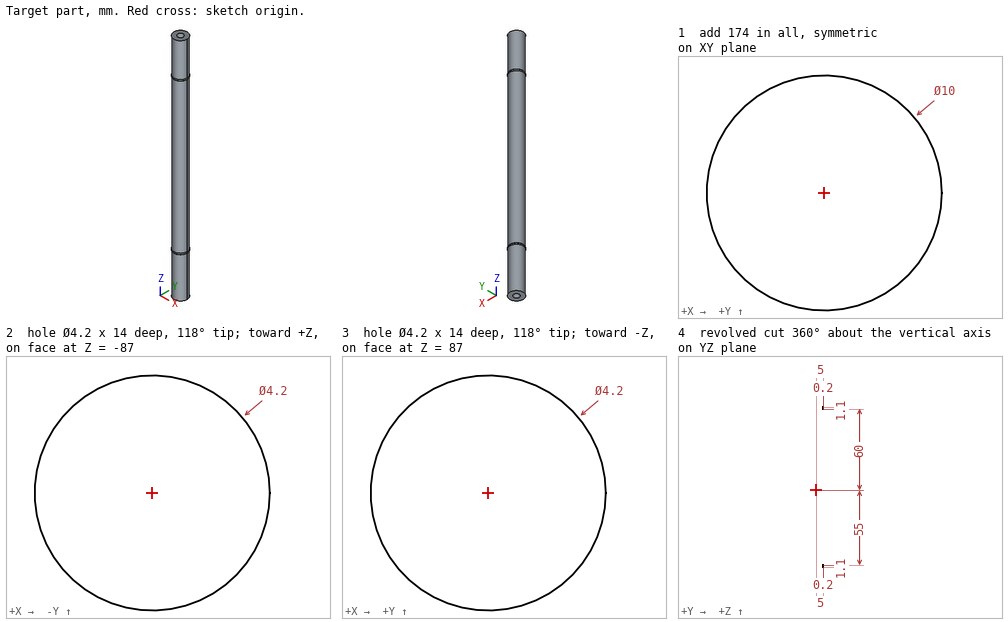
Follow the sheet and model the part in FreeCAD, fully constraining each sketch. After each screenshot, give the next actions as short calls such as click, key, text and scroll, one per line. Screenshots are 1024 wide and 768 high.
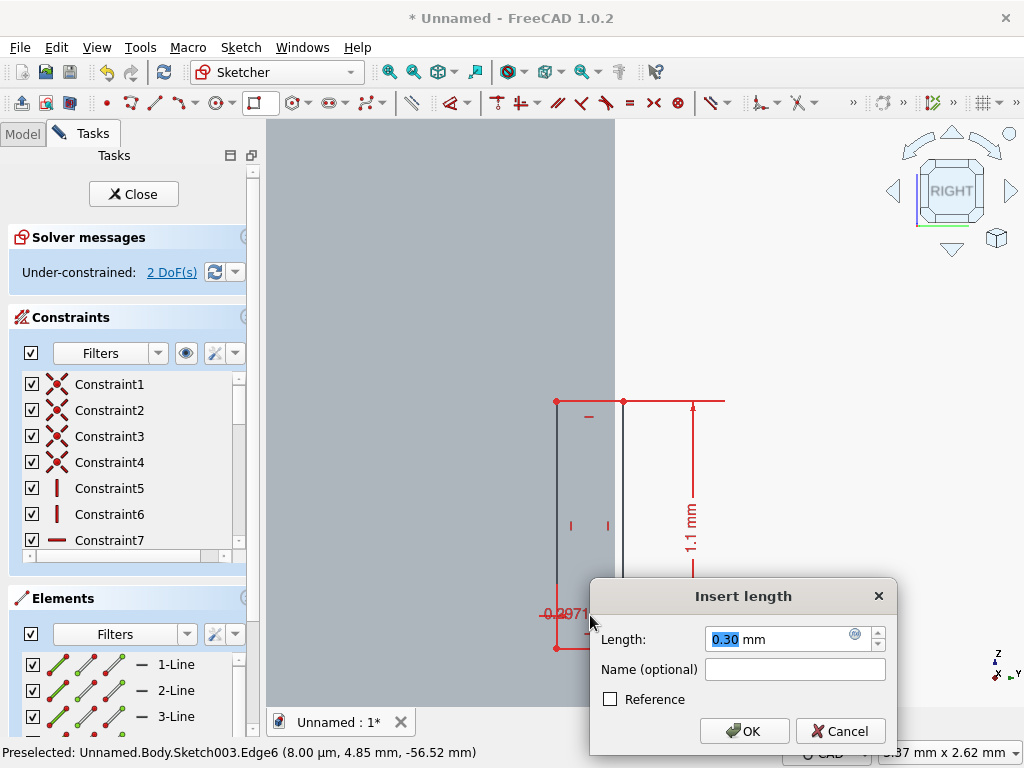
text(0.2)
key(Return)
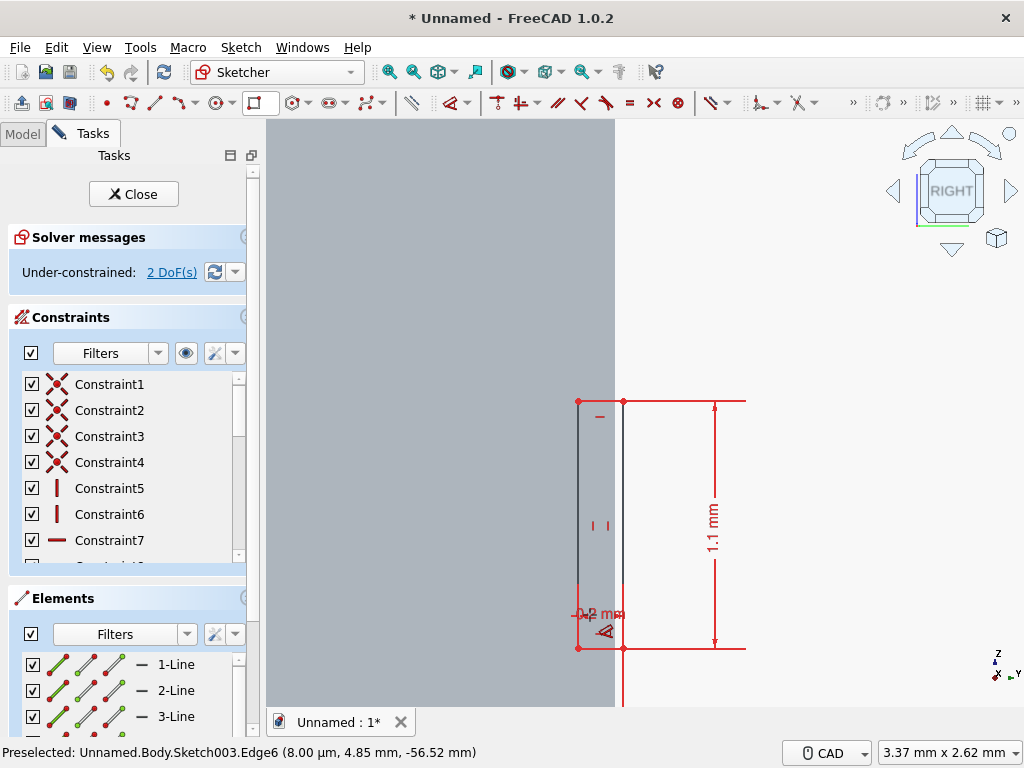
scroll(576, 413, down, 15)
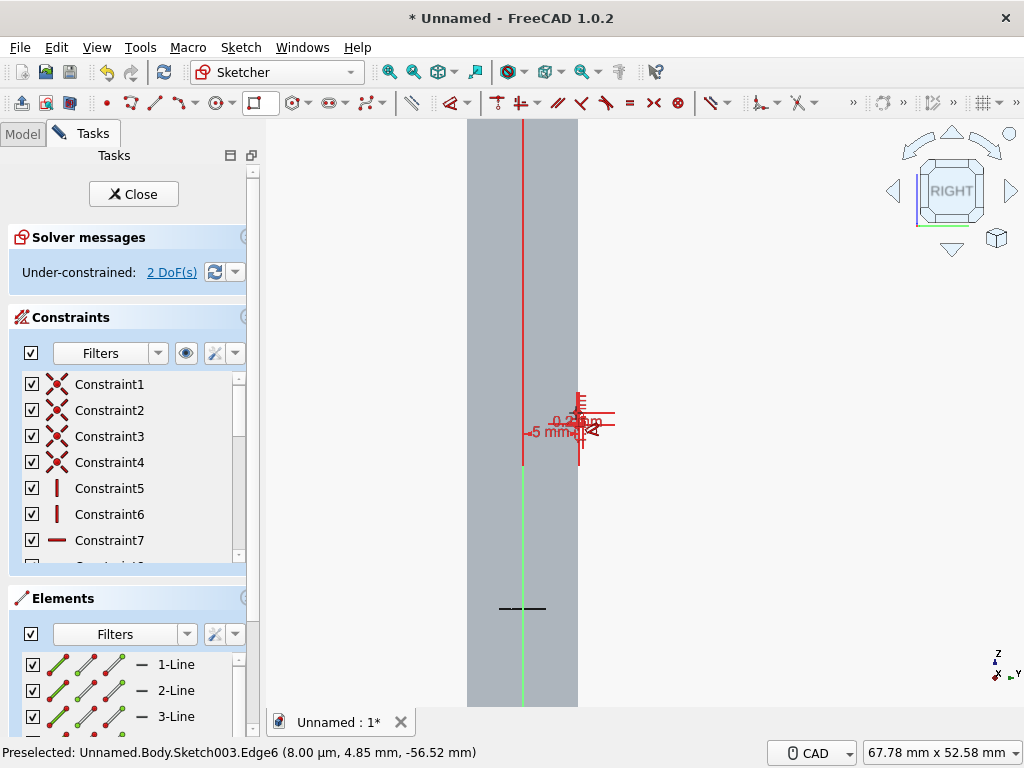
scroll(588, 679, down, 6)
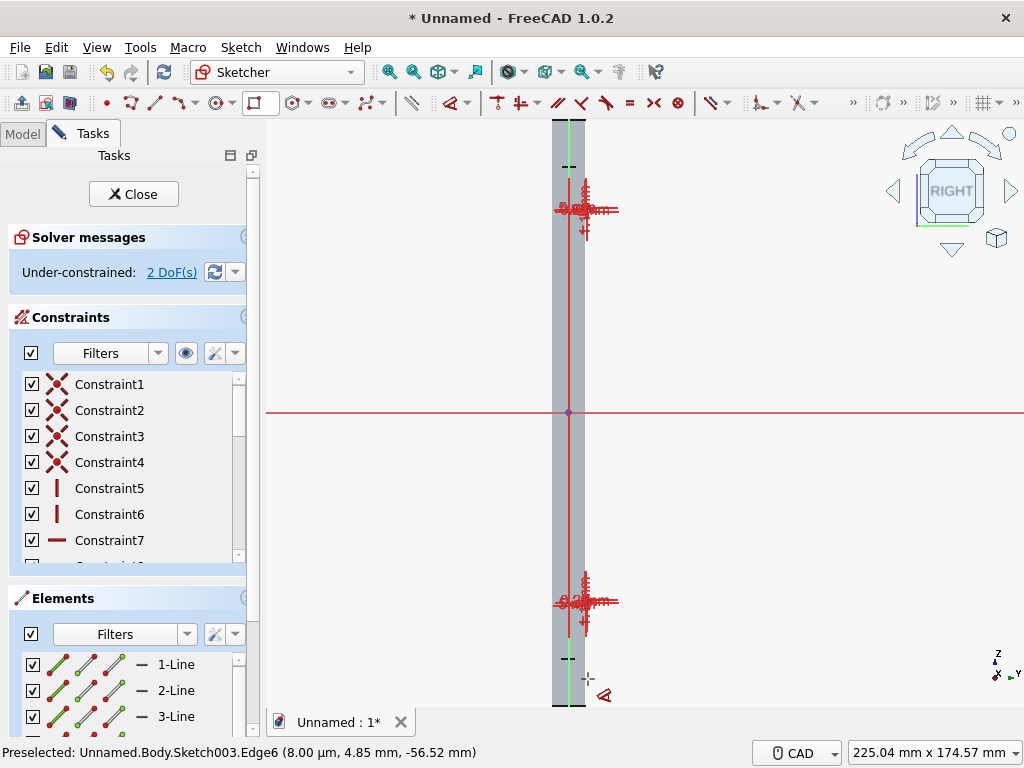
scroll(585, 212, up, 14)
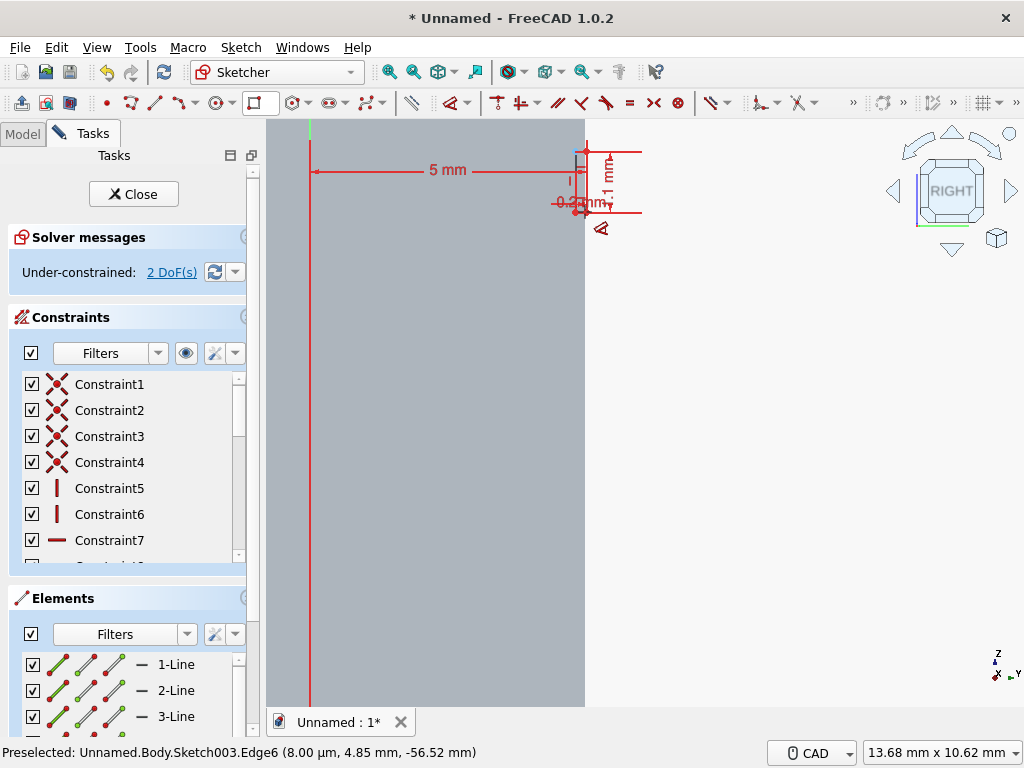
click(576, 213)
click(610, 446)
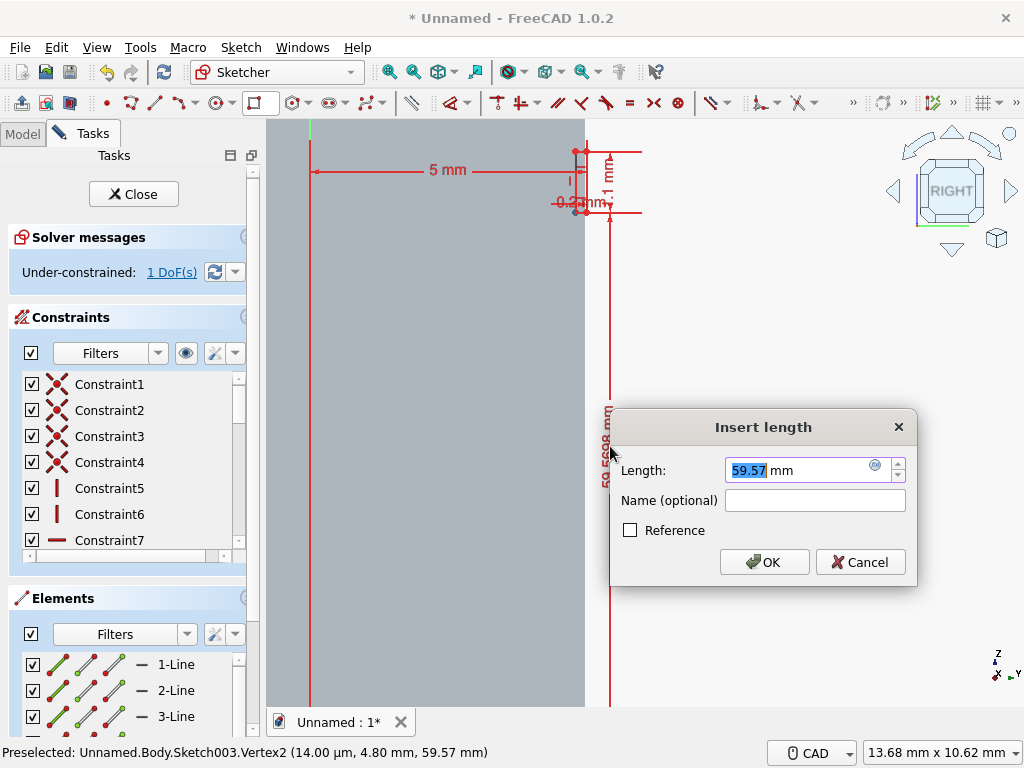
text(60)
key(Return)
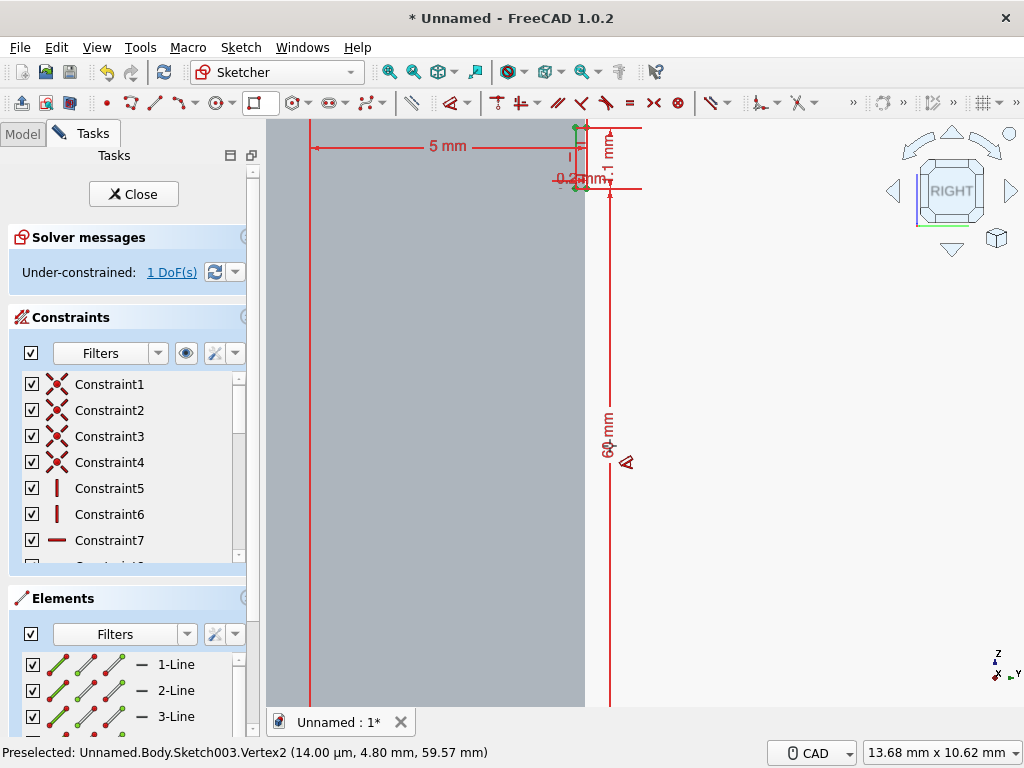
scroll(585, 221, down, 14)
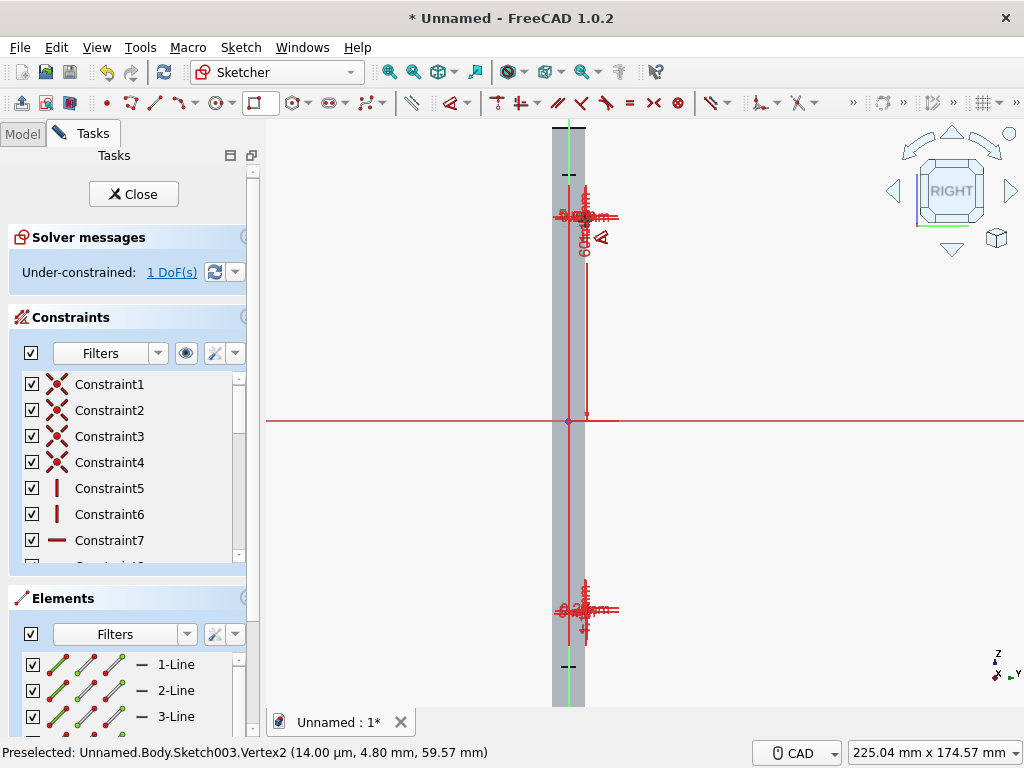
scroll(585, 608, up, 14)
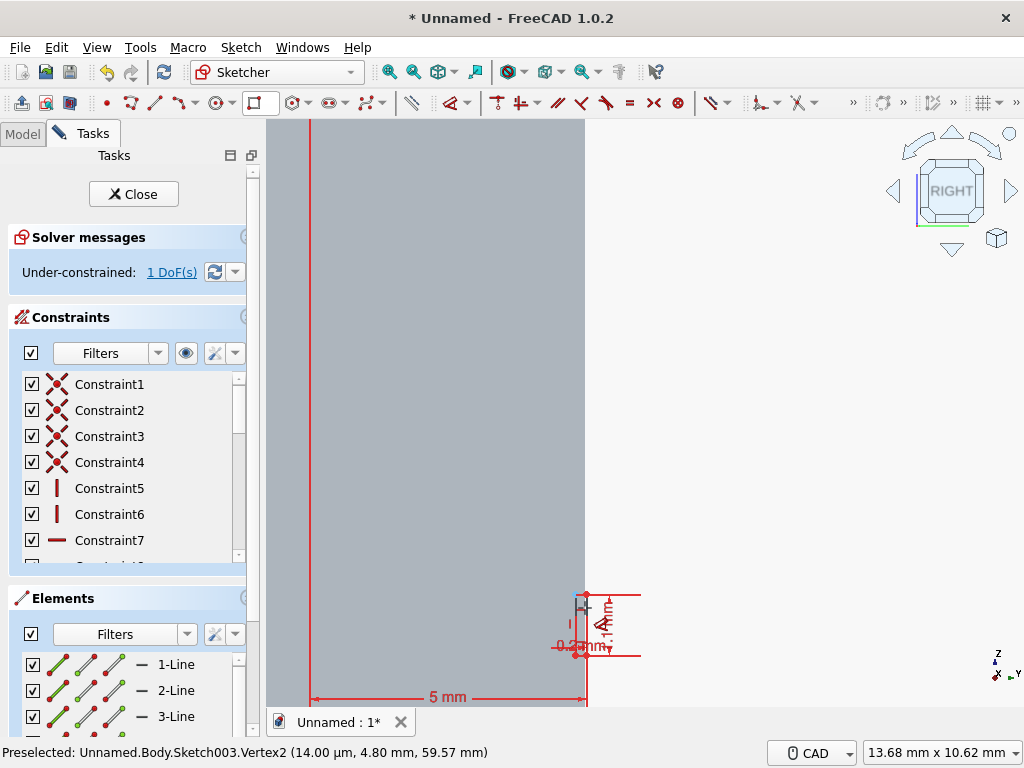
click(576, 595)
click(610, 371)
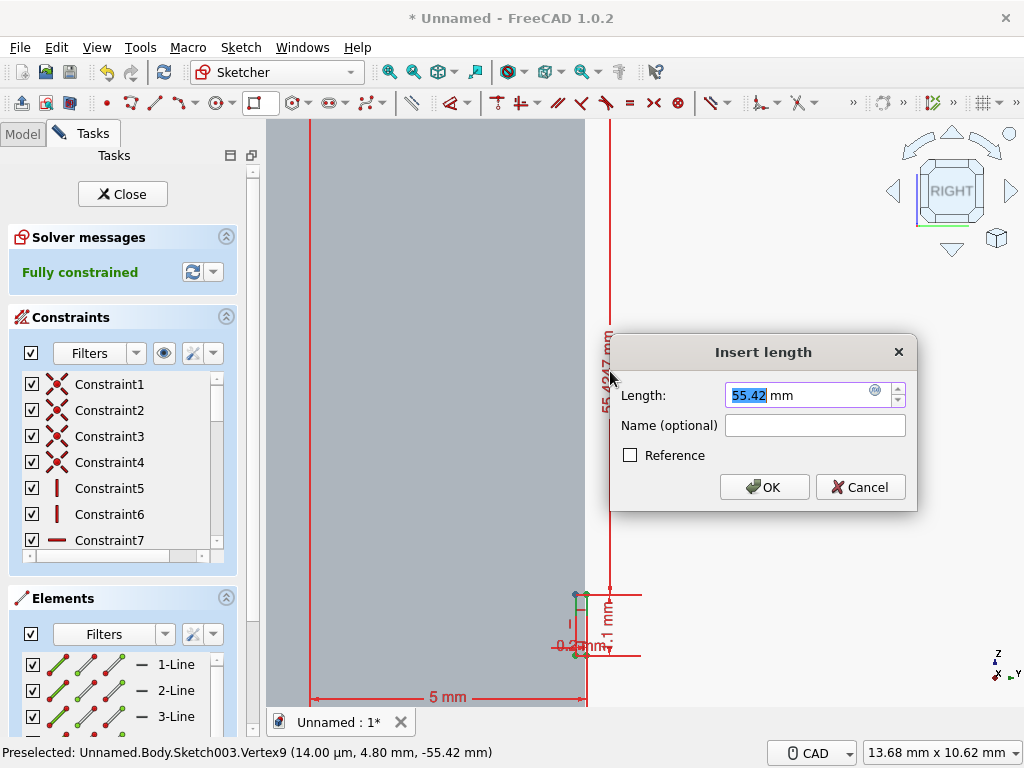
text(55)
key(Return)
key(Escape)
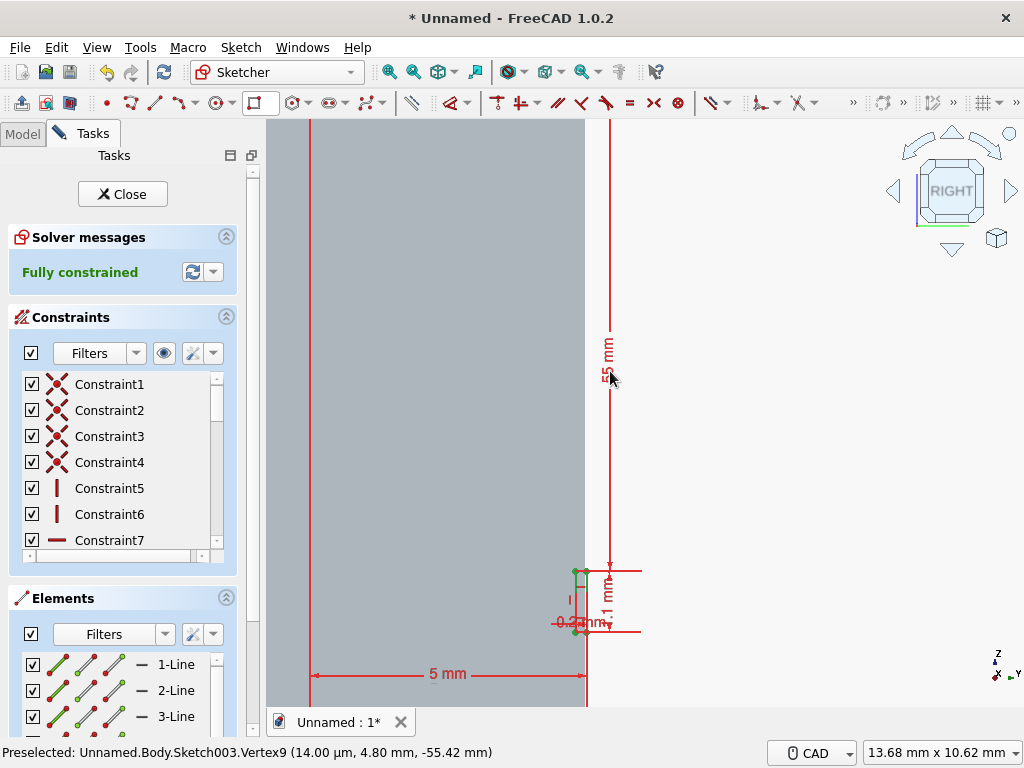
click(123, 194)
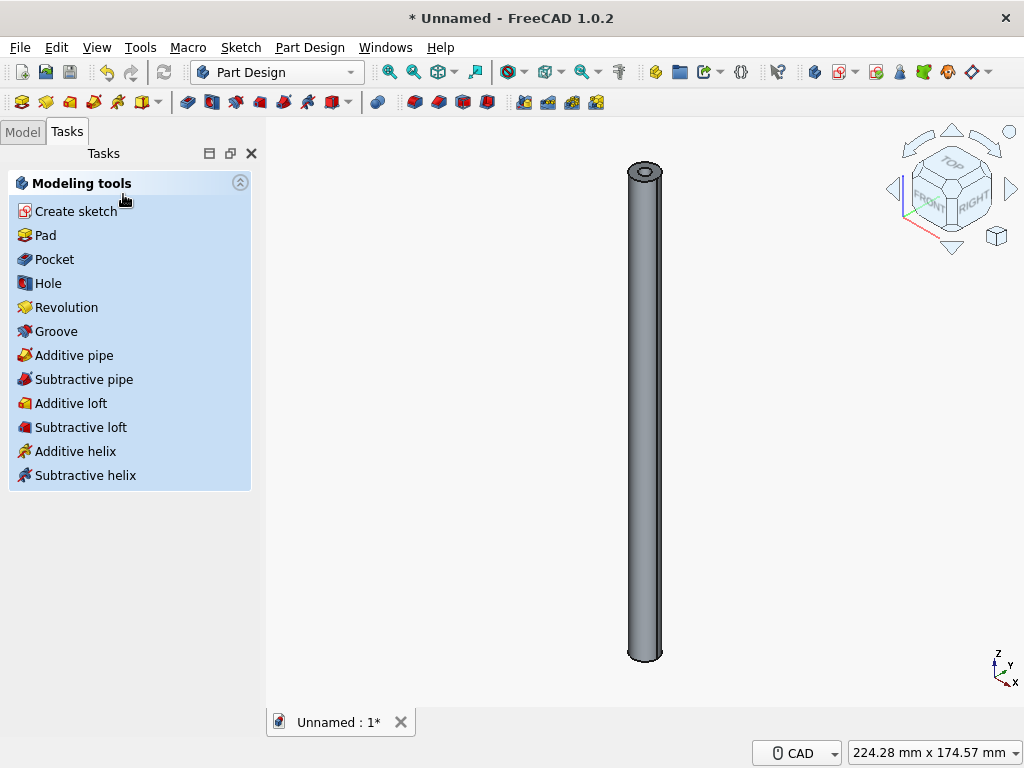
click(236, 102)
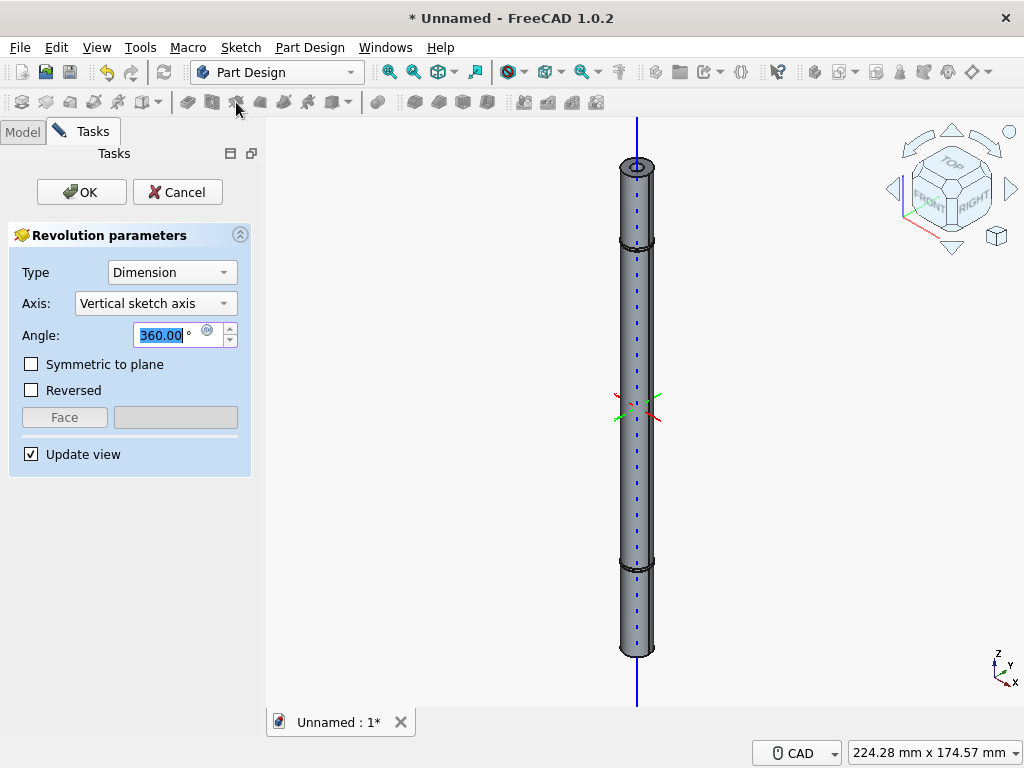
click(82, 192)